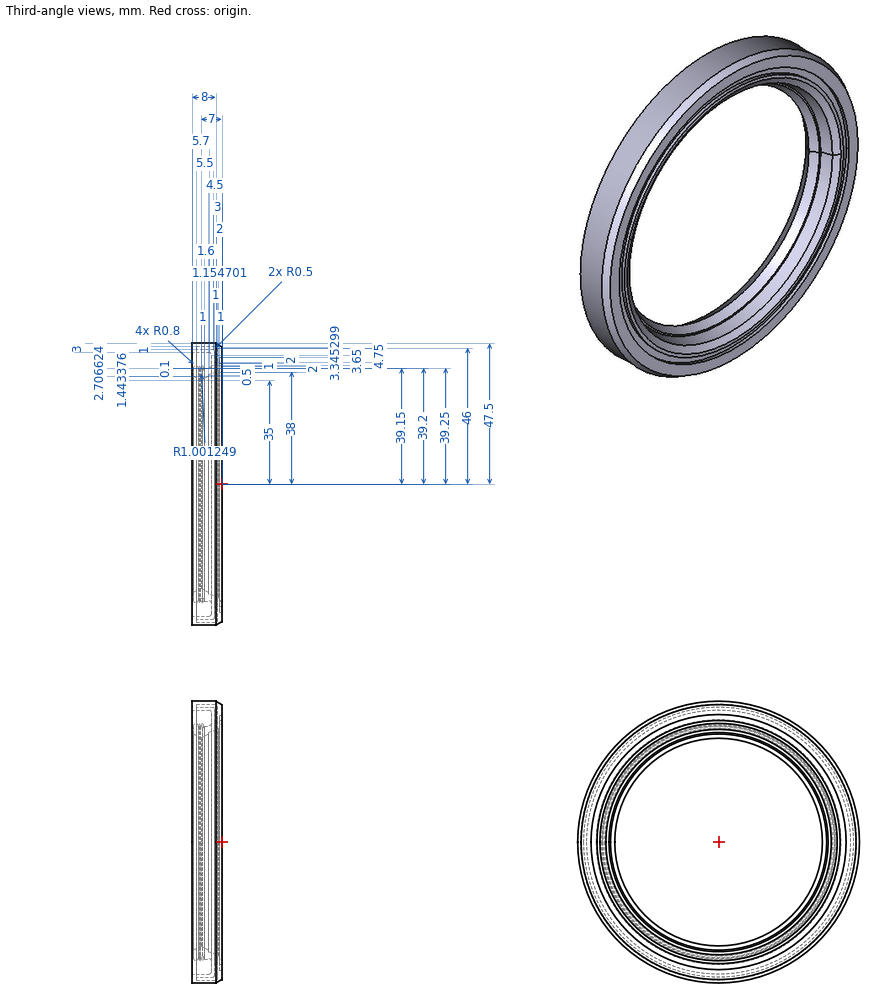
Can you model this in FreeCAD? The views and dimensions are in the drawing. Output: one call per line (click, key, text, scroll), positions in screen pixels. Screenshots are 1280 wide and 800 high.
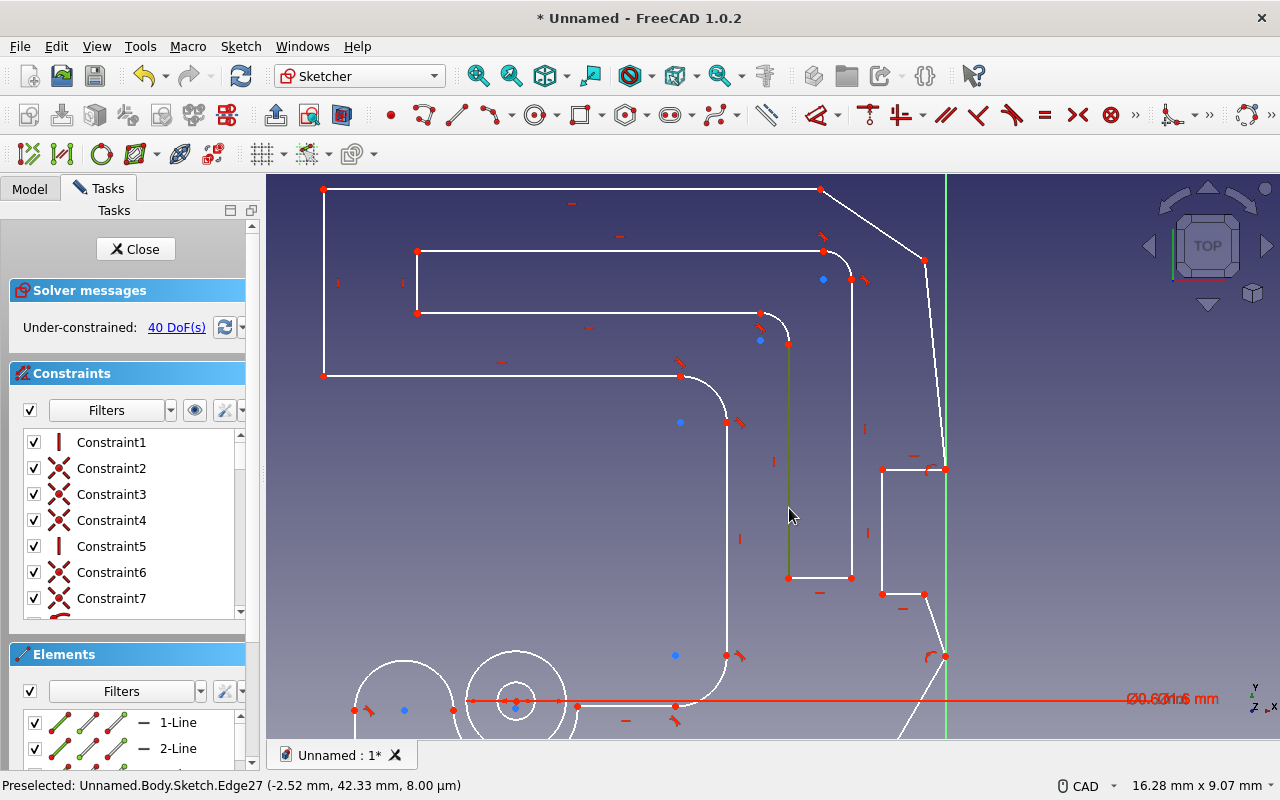
click(787, 331)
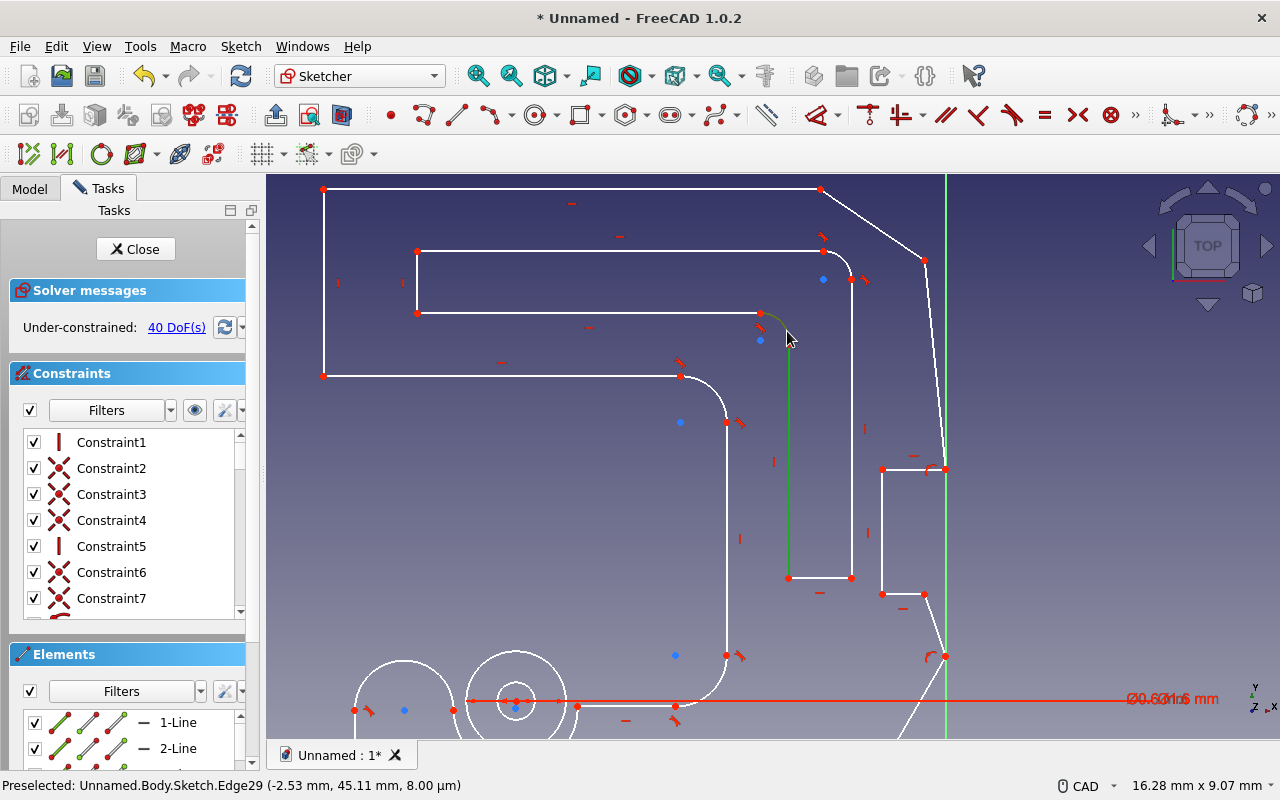
click(1012, 116)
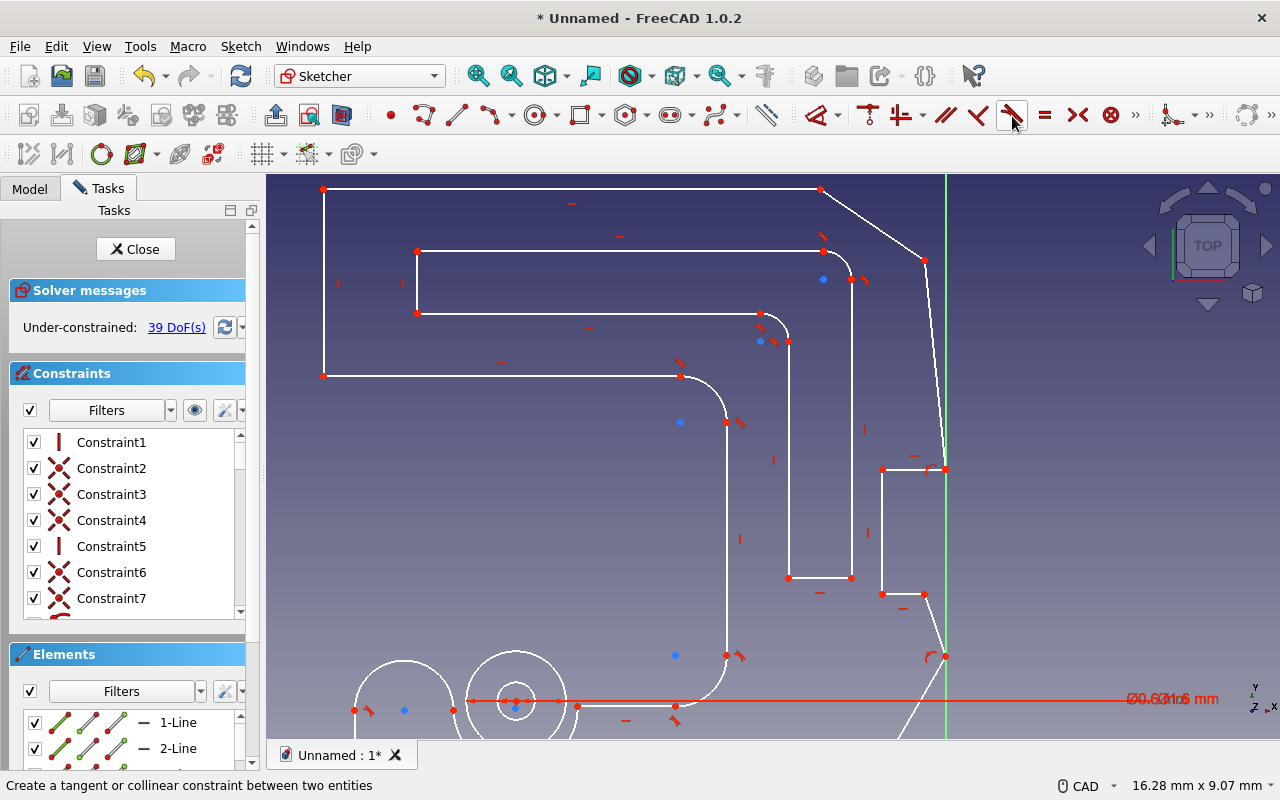
click(931, 613)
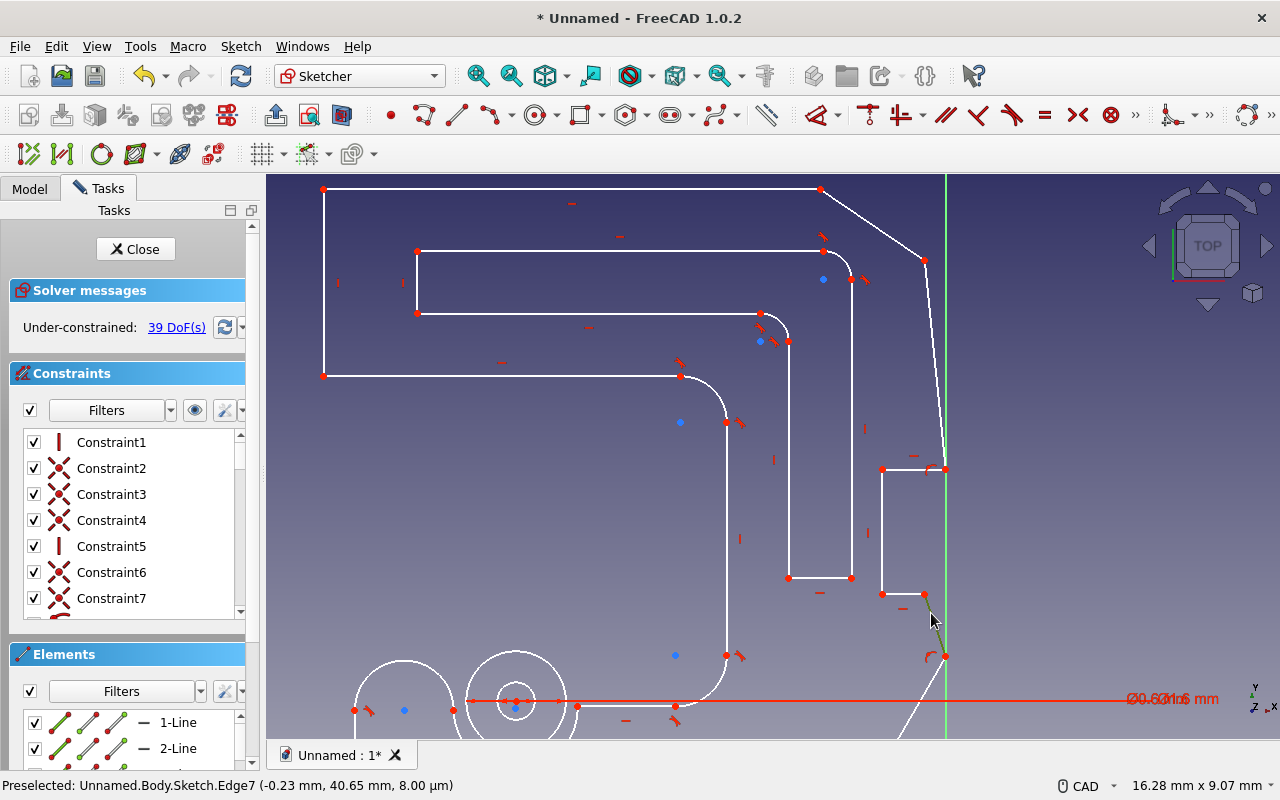
key(v)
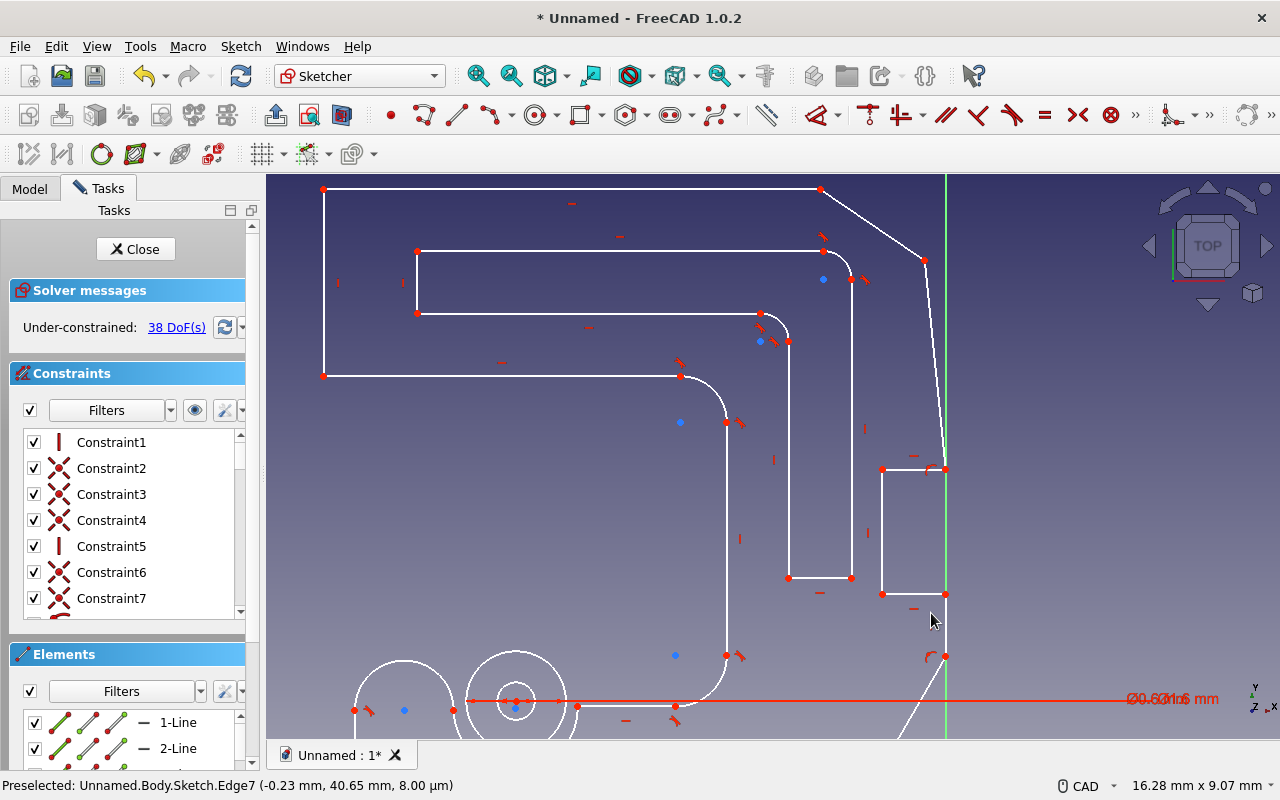
click(931, 323)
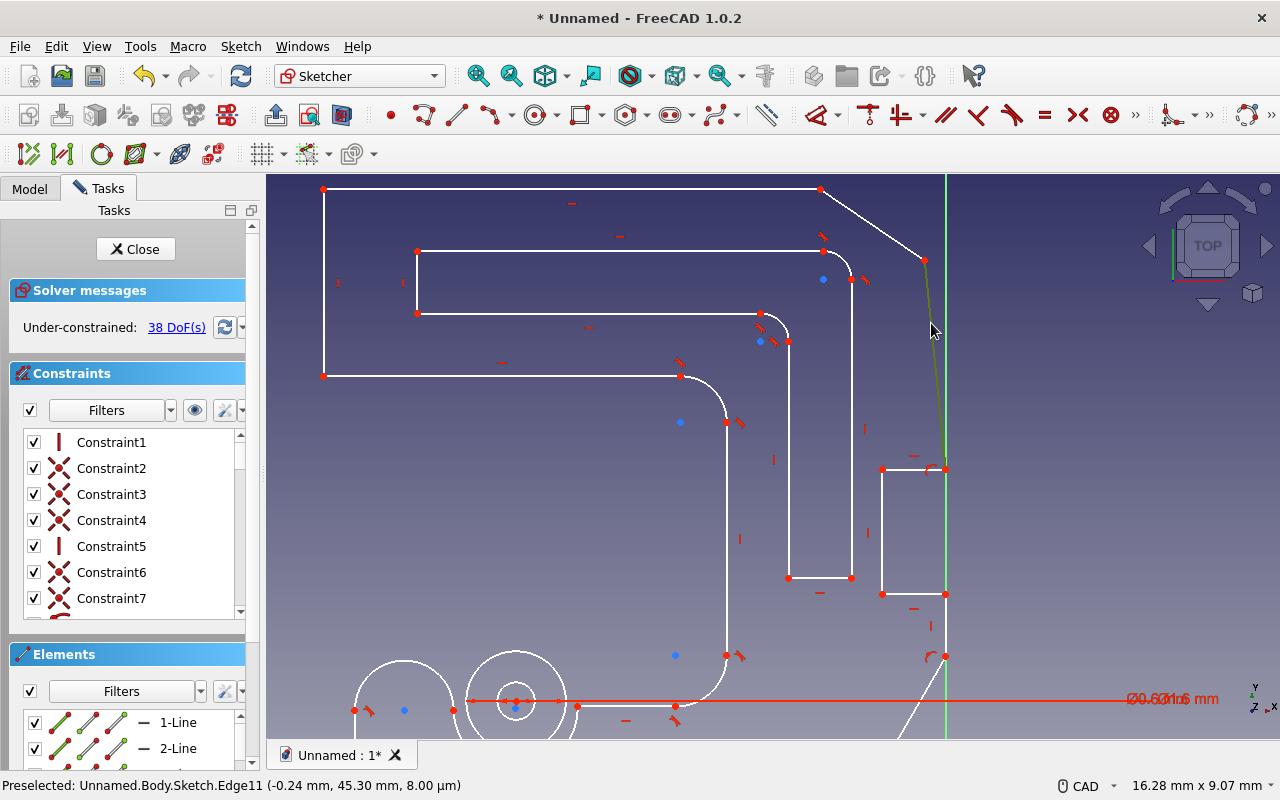
click(922, 116)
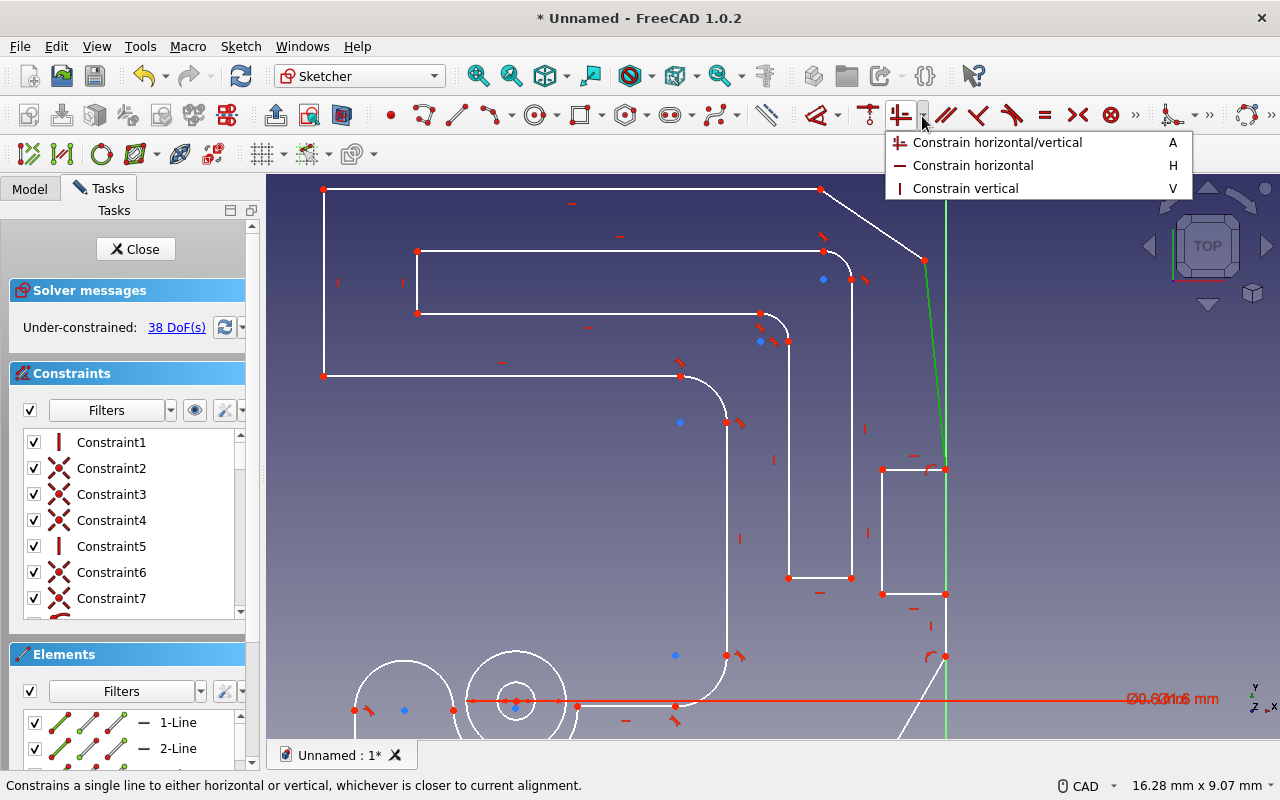
click(1039, 188)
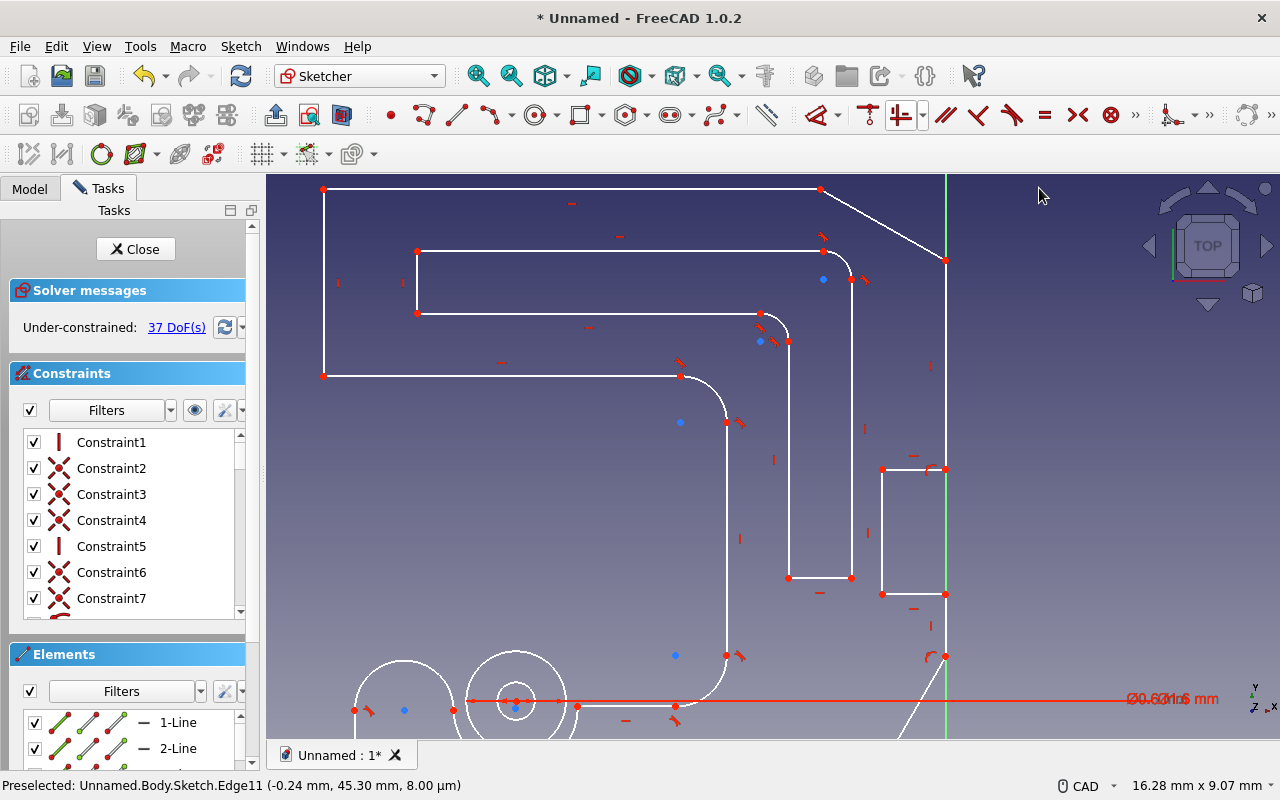
click(722, 401)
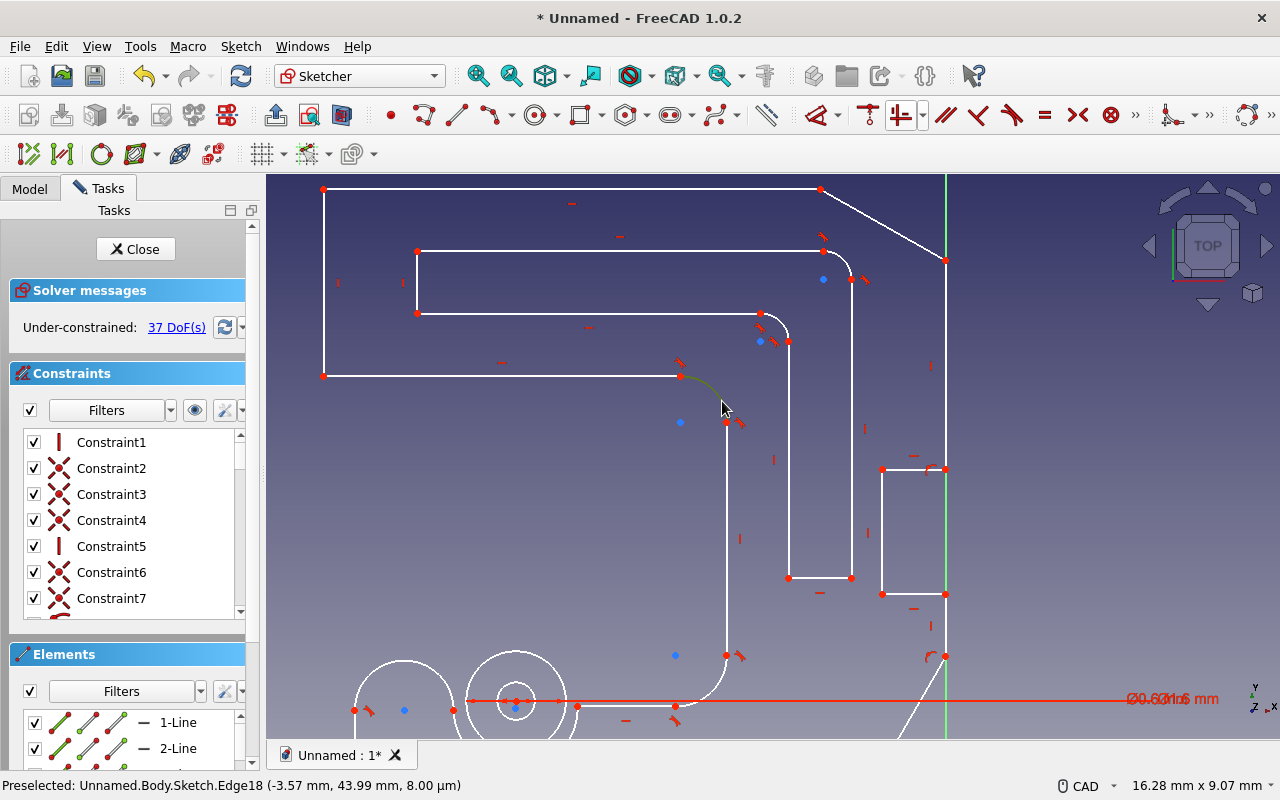
click(699, 701)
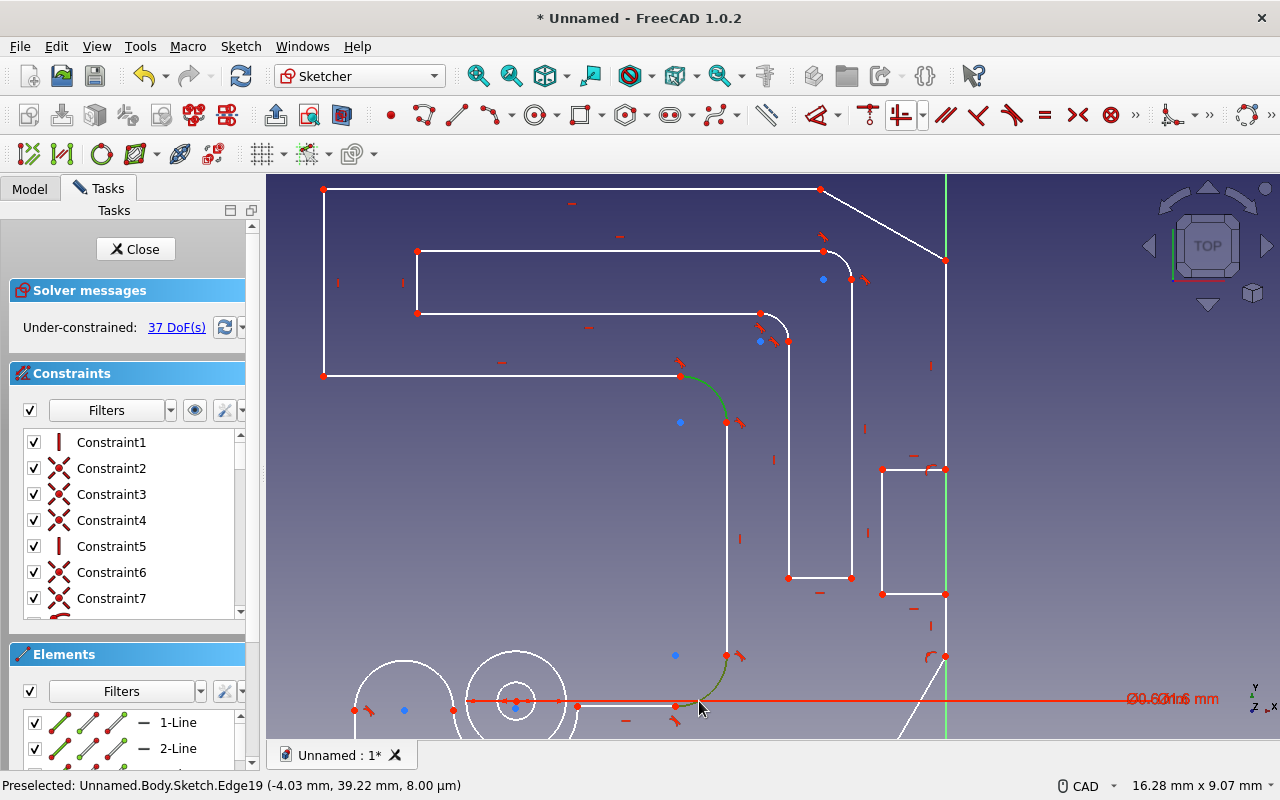
click(434, 670)